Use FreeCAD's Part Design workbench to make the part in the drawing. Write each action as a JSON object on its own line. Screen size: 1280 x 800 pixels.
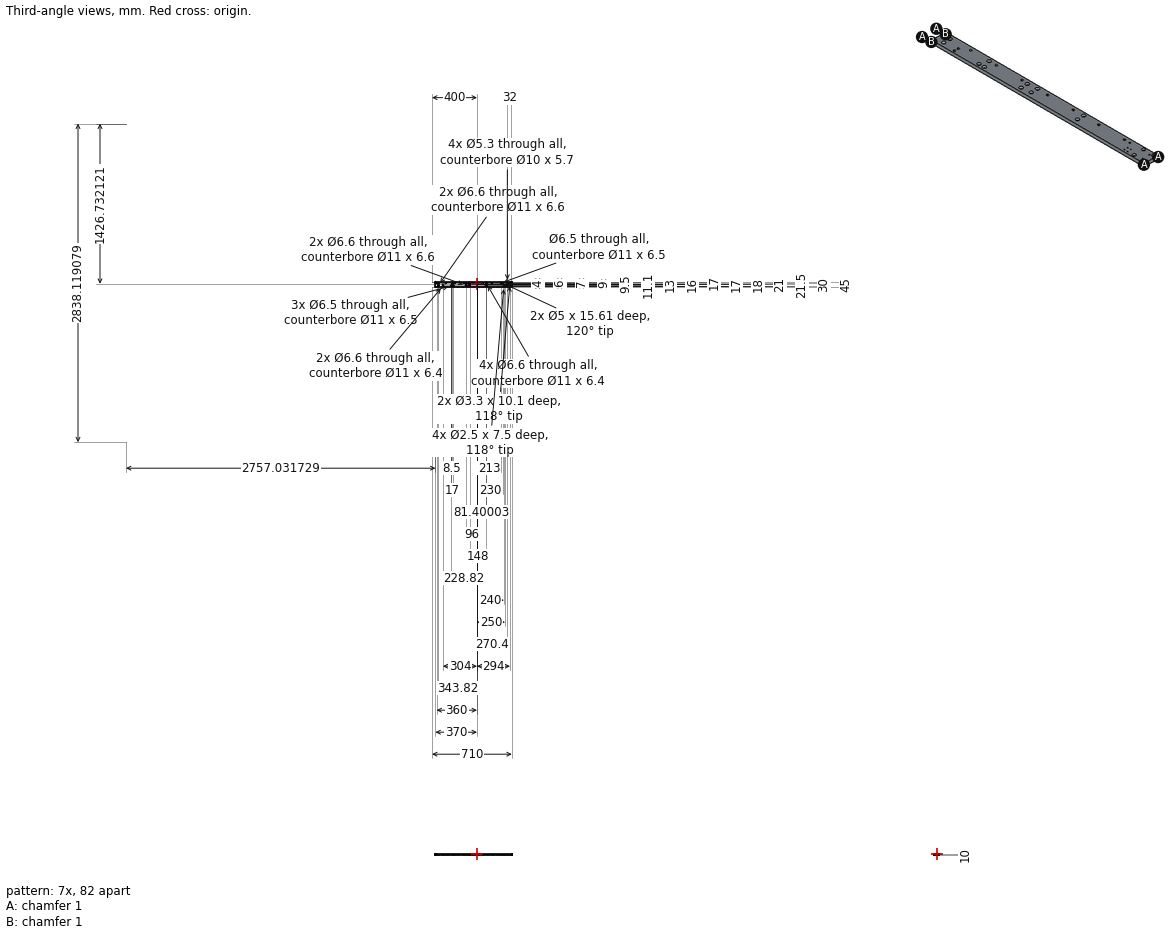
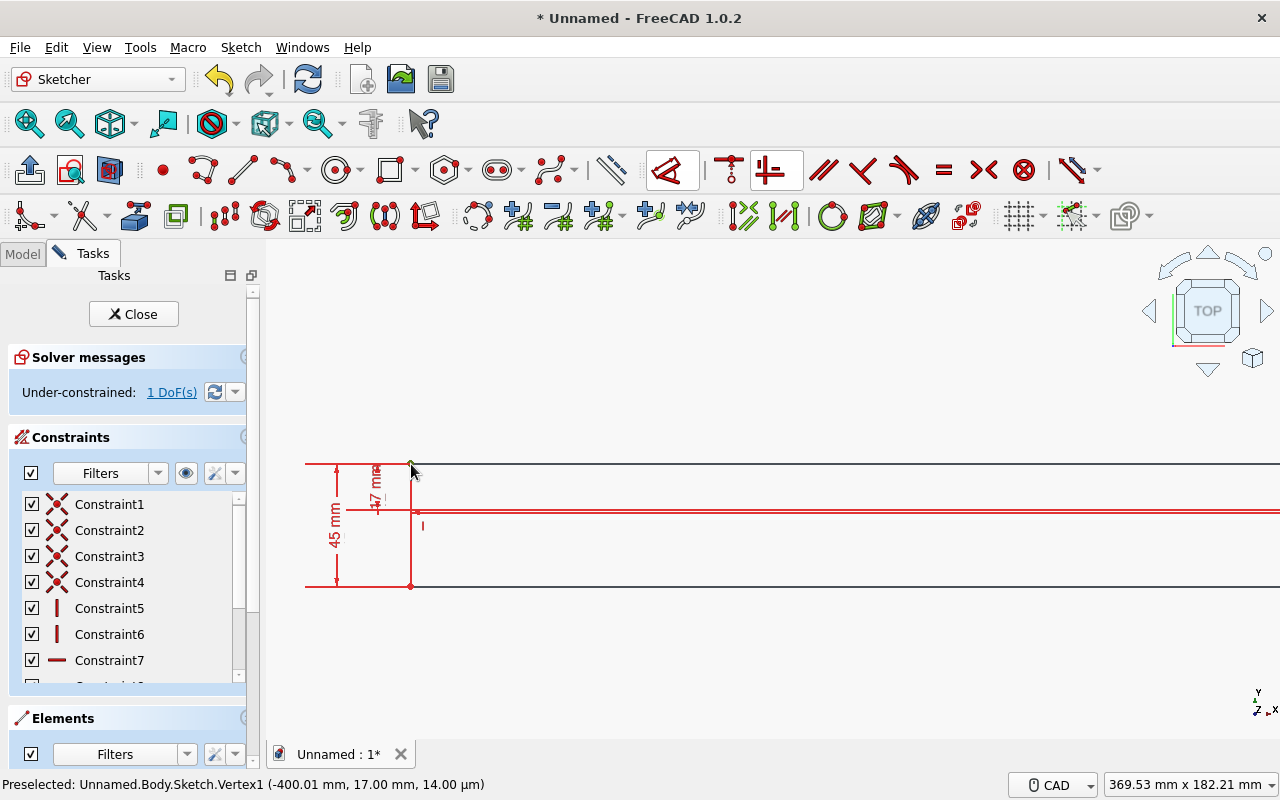
{"action": "key", "text": "l"}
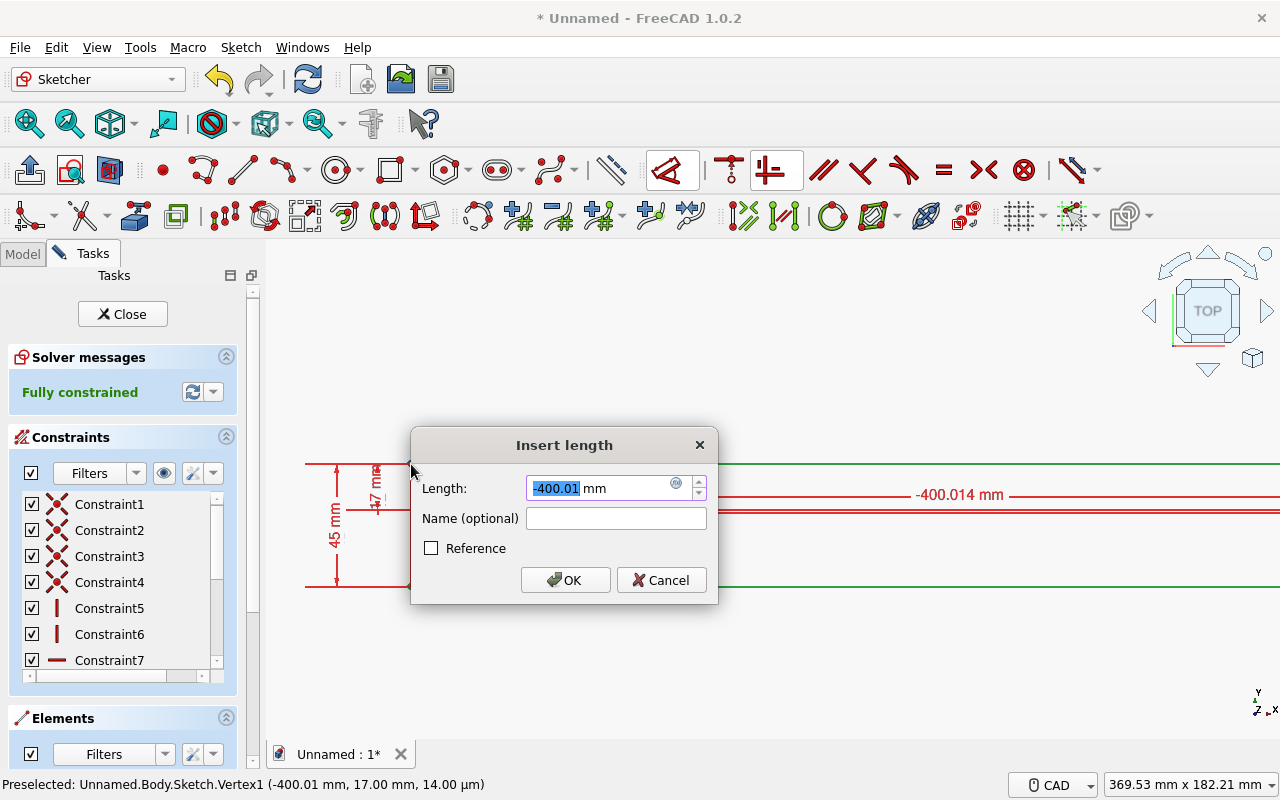
{"action": "type", "text": "-400"}
{"action": "key", "text": "Return"}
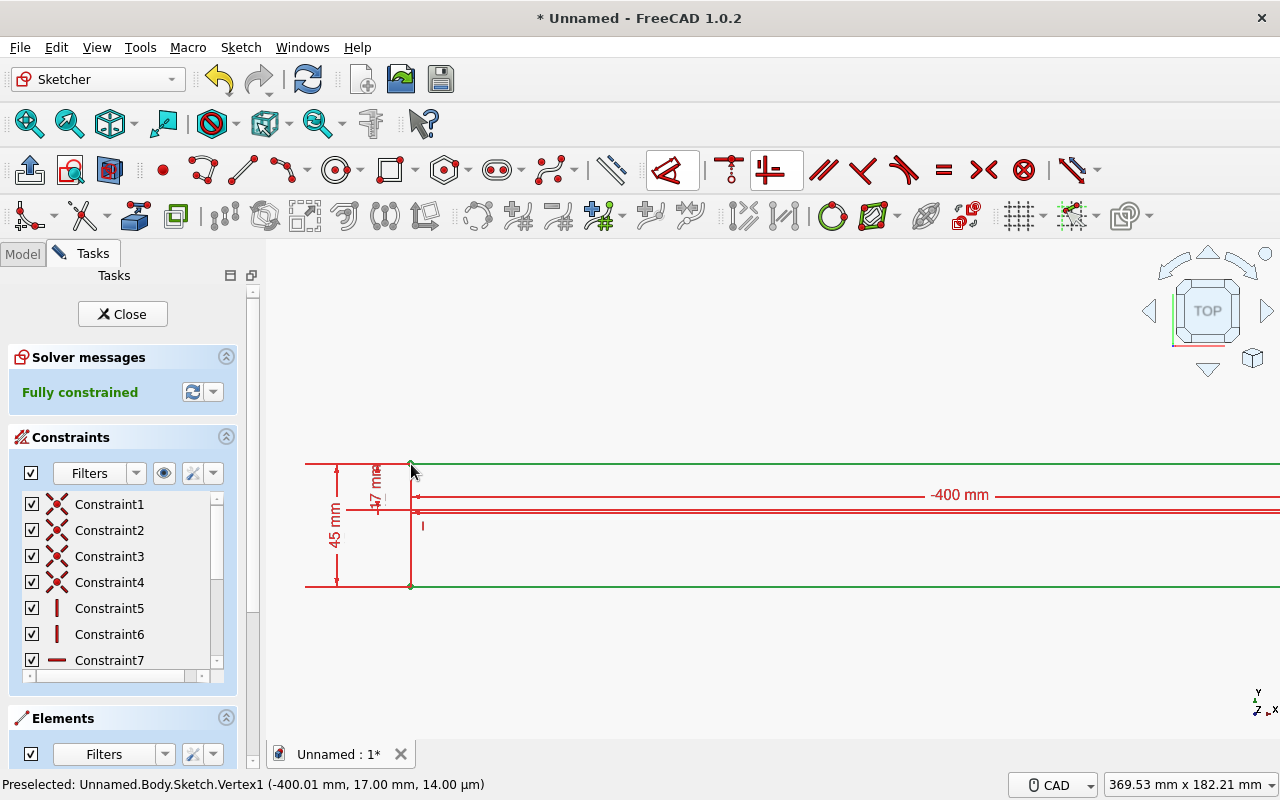
{"action": "left_click", "coordinate": [123, 314]}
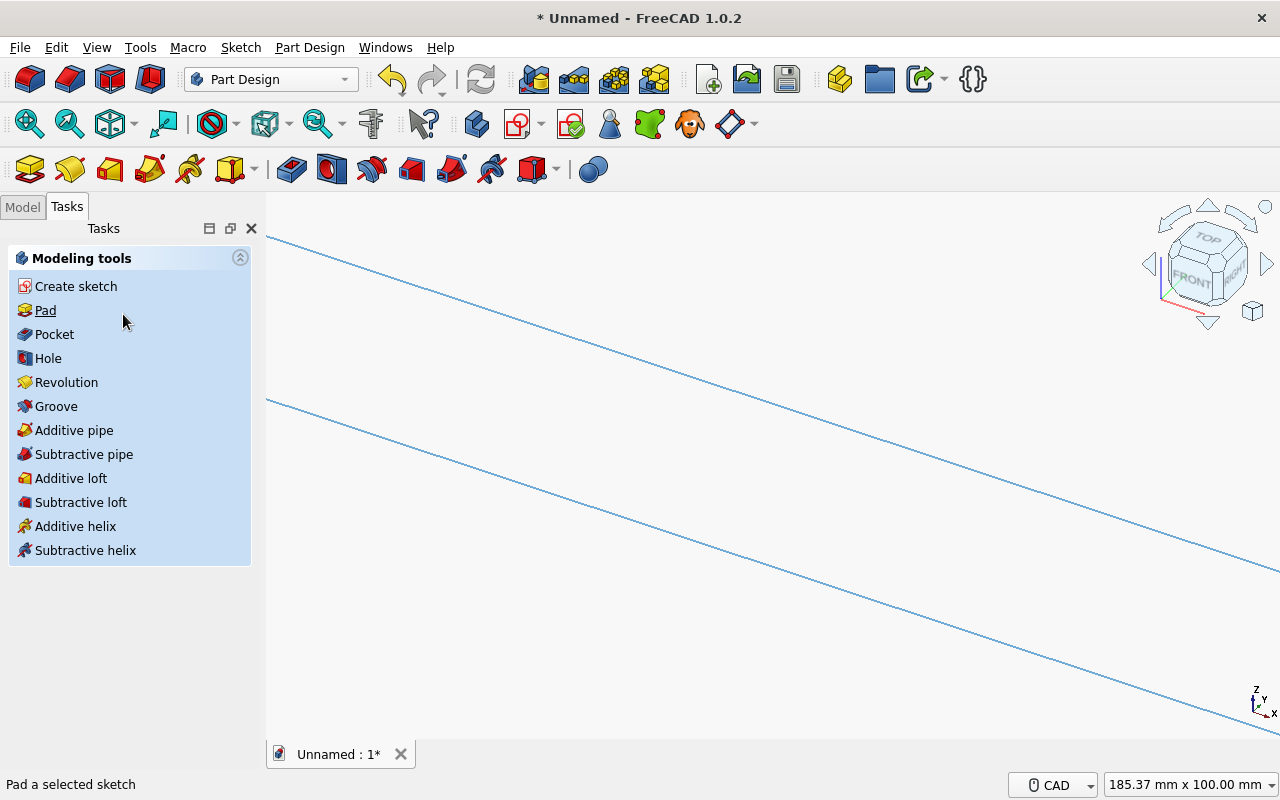
{"action": "left_click", "coordinate": [30, 170]}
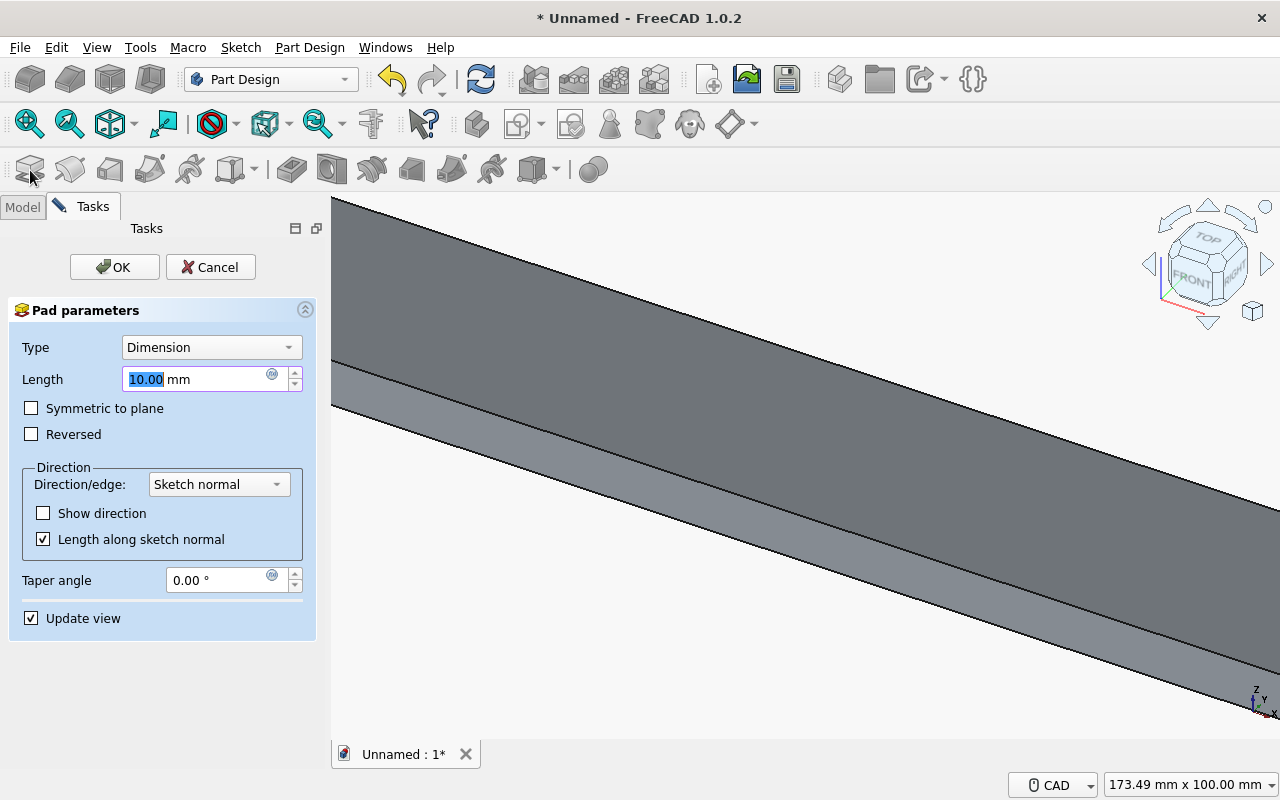
{"action": "type", "text": "10"}
{"action": "key", "text": "Tab"}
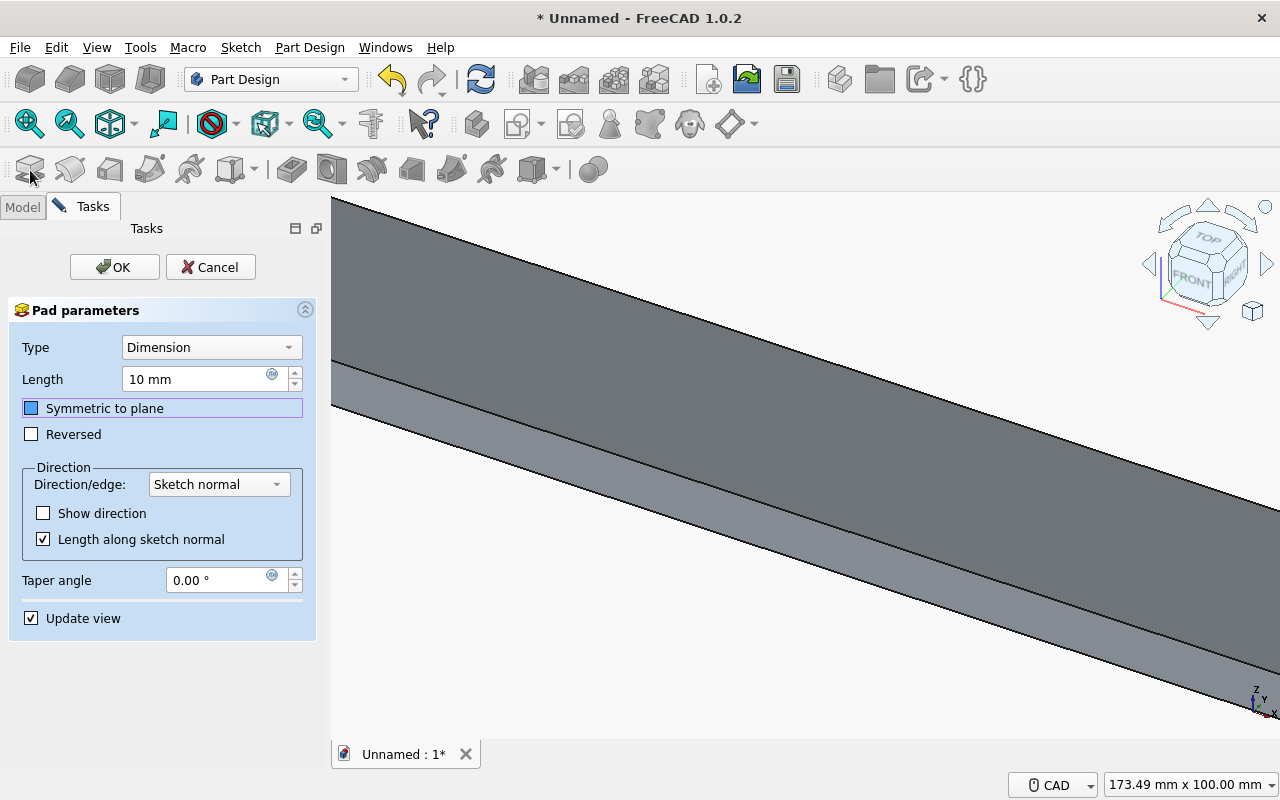
{"action": "left_click", "coordinate": [30, 434]}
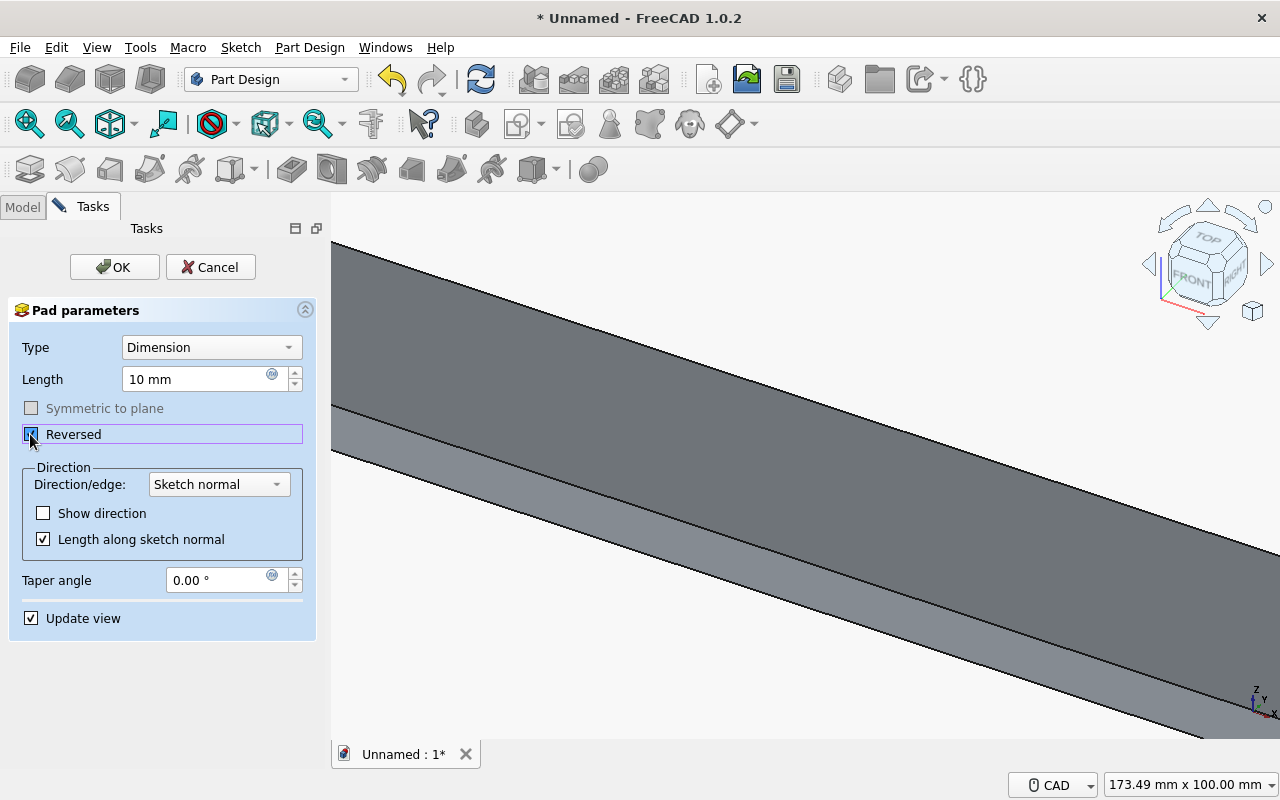
{"action": "left_click", "coordinate": [115, 267]}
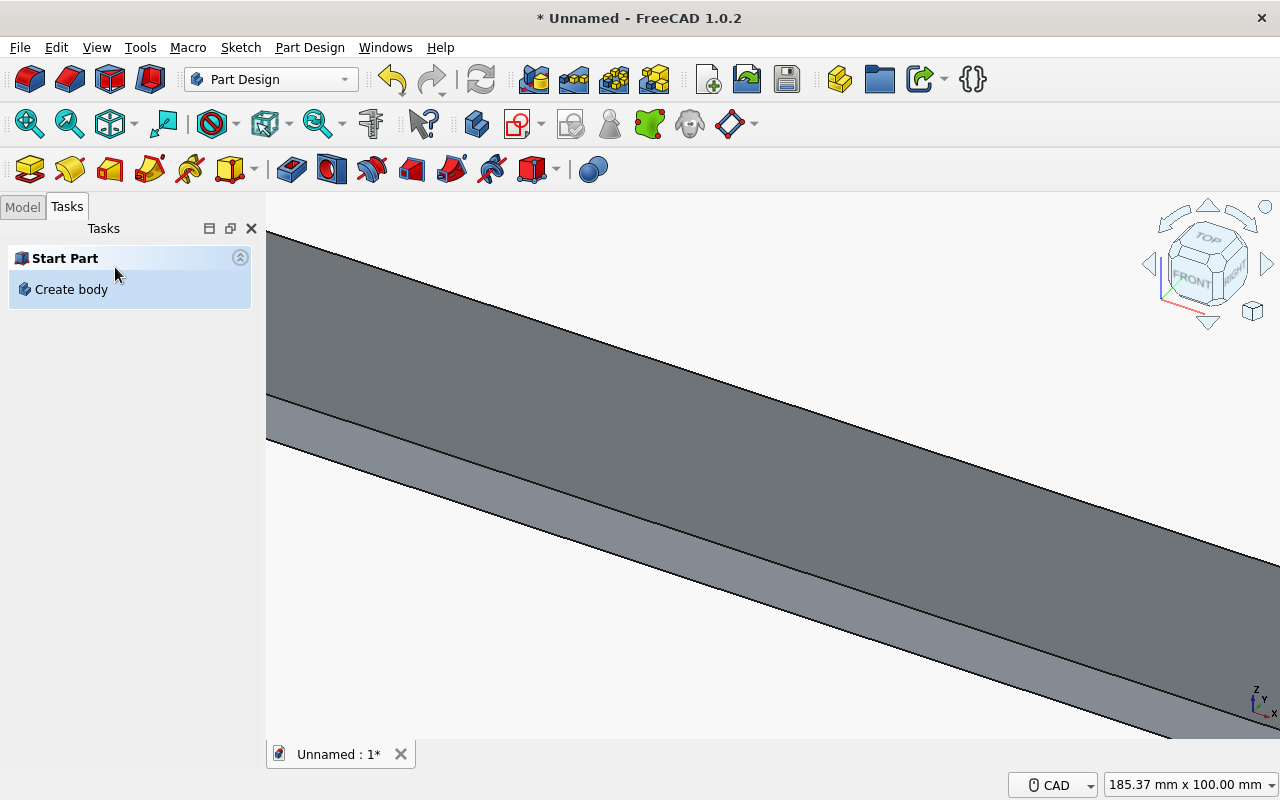
{"action": "left_click", "coordinate": [30, 124]}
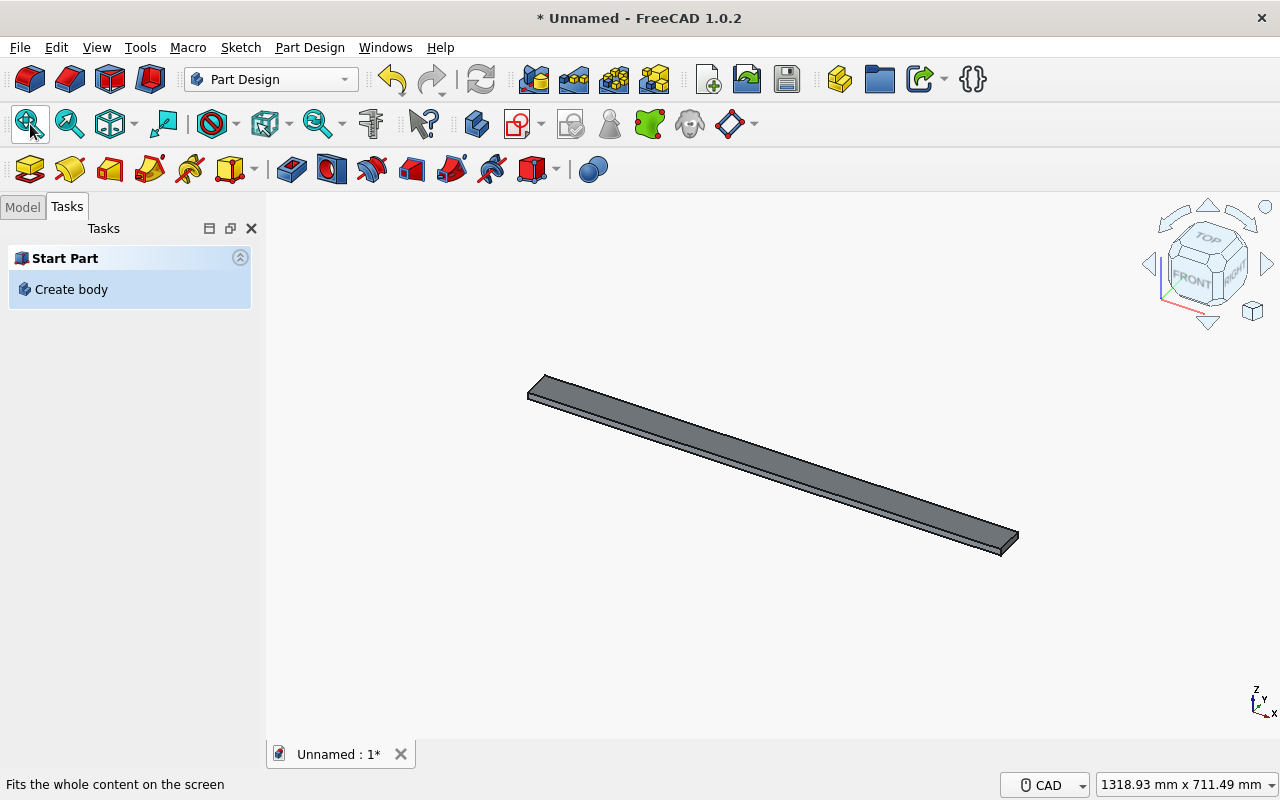
{"action": "key", "text": "5"}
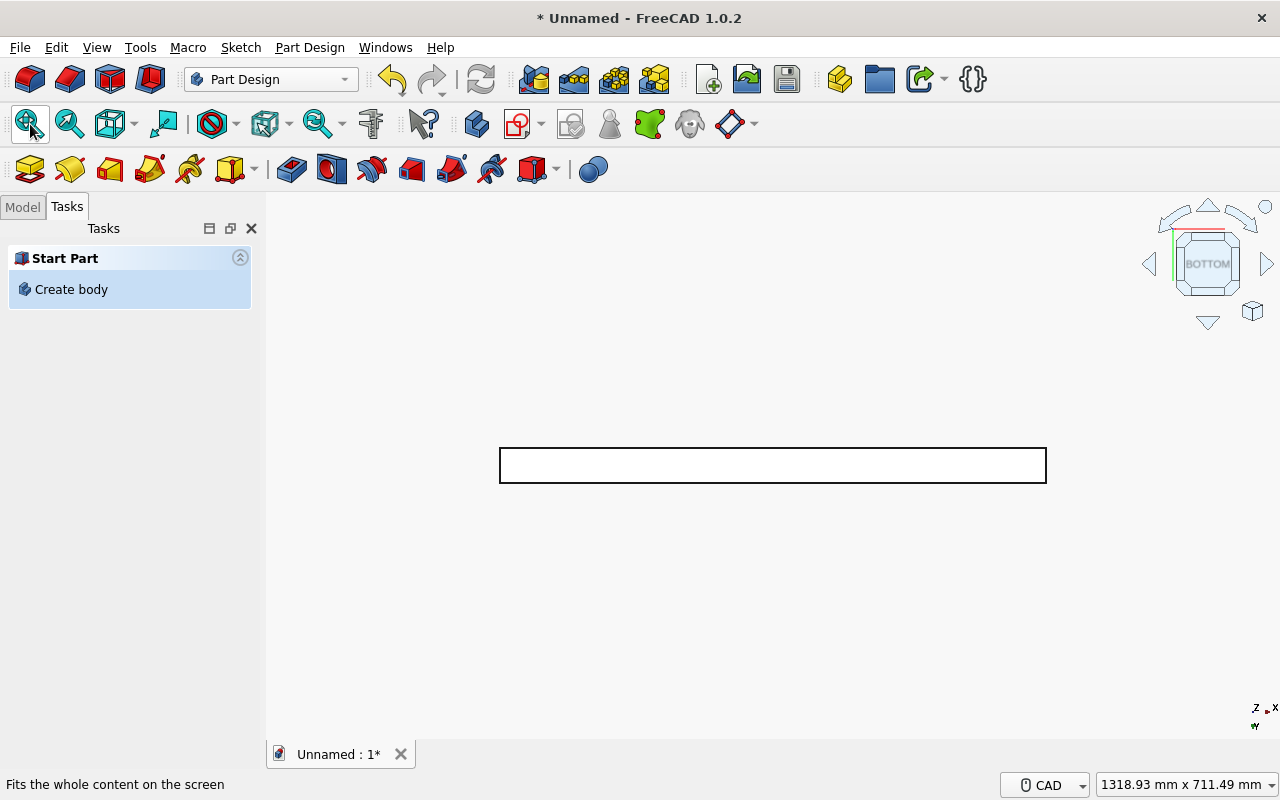
{"action": "left_click", "coordinate": [1007, 464]}